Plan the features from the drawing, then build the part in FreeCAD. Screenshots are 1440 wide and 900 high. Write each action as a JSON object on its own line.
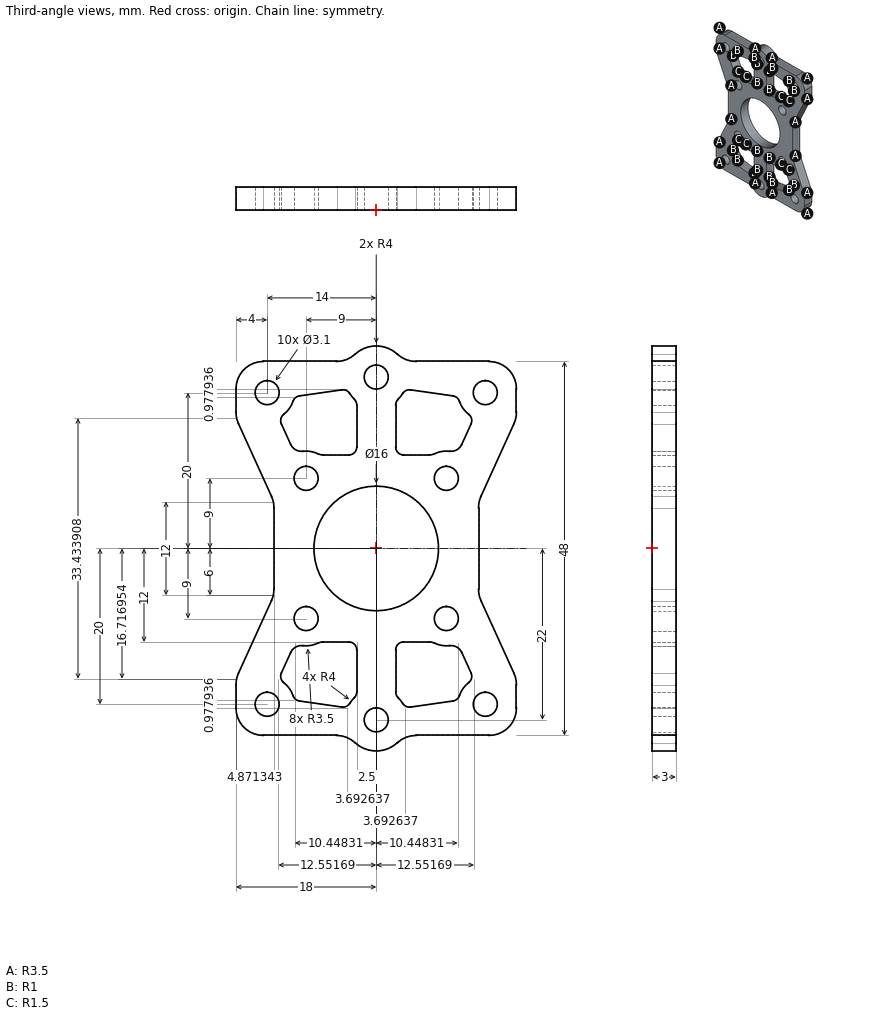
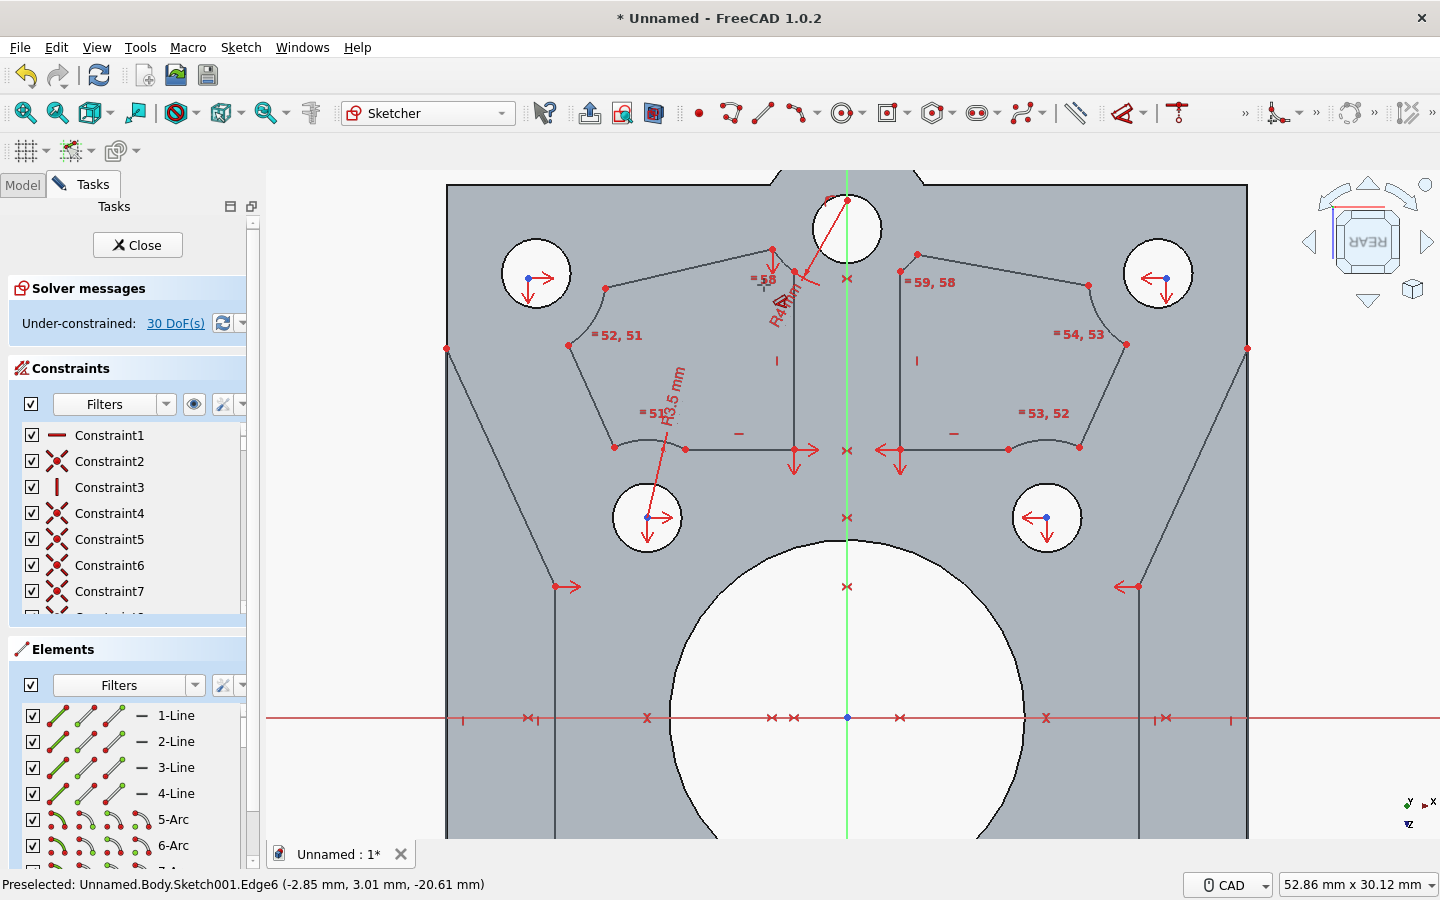
{"action": "left_click", "coordinate": [555, 774]}
{"action": "left_click", "coordinate": [521, 699]}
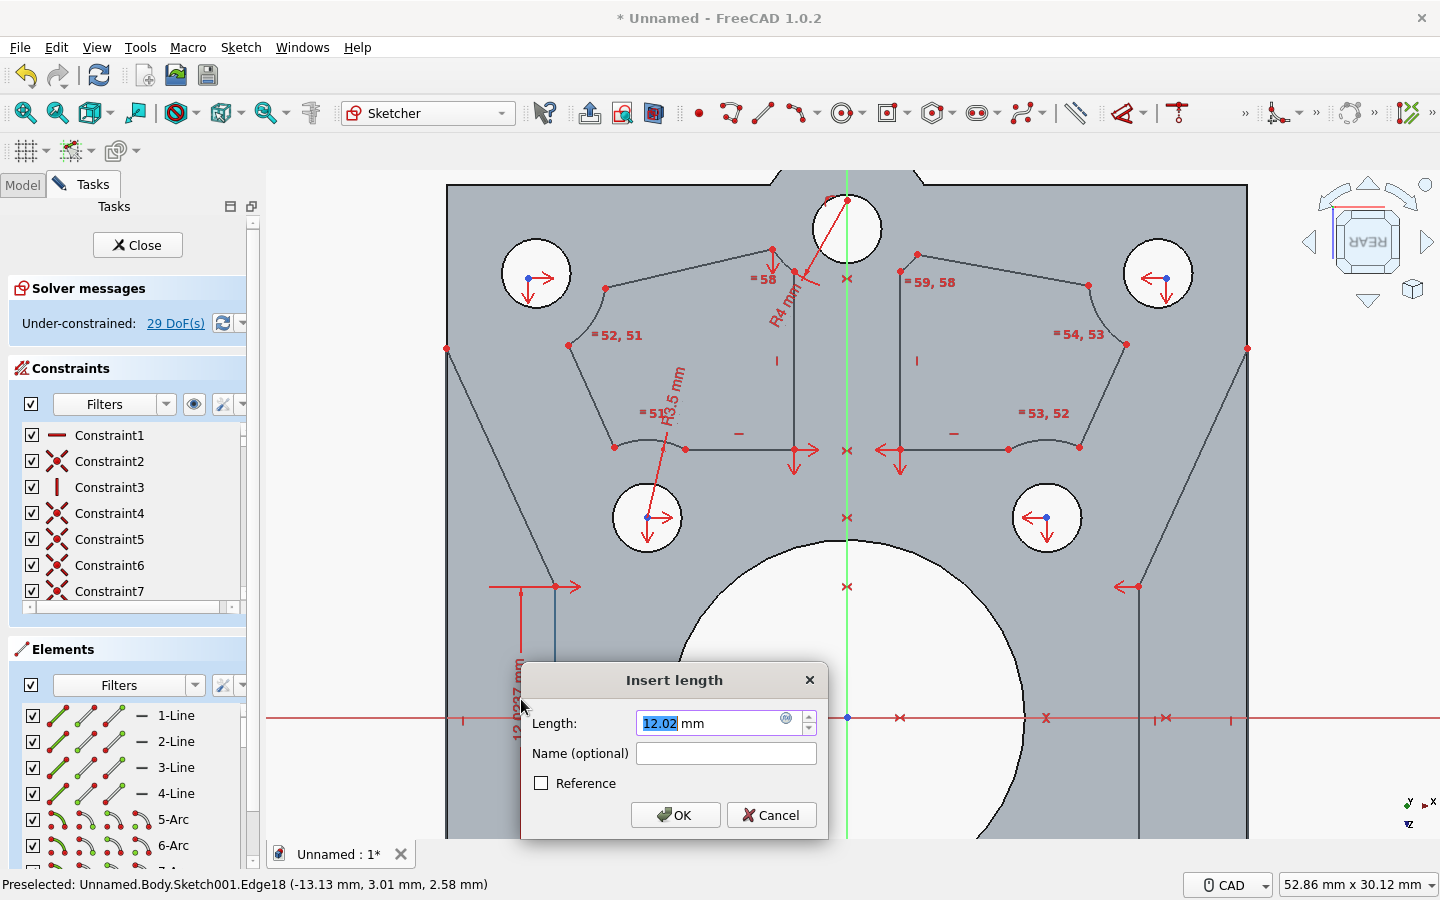
{"action": "type", "text": "12"}
{"action": "key", "text": "Return"}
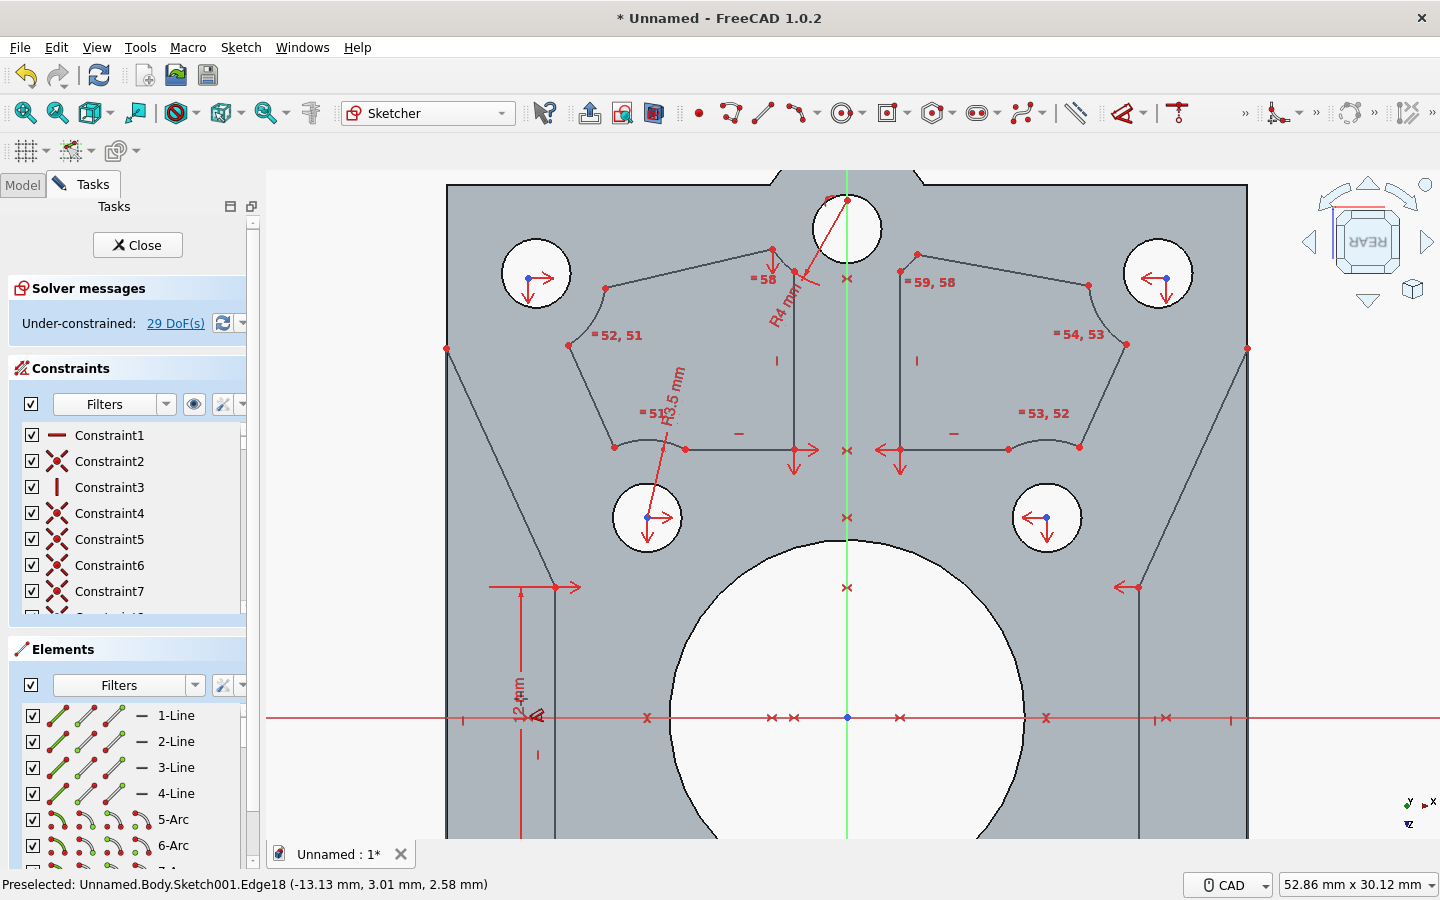
{"action": "left_click", "coordinate": [1139, 667]}
{"action": "left_click", "coordinate": [1173, 699]}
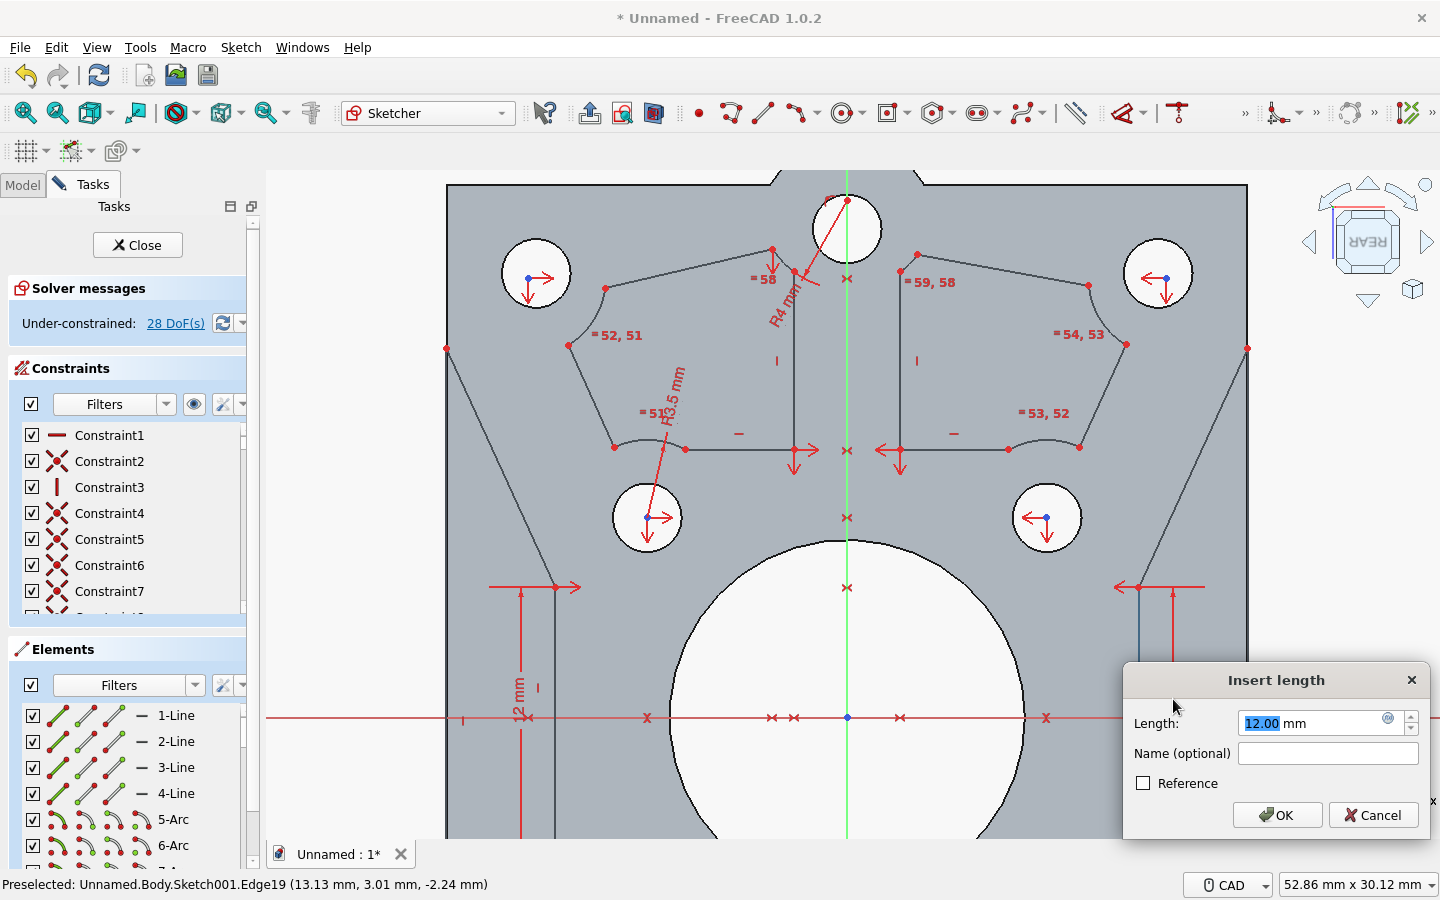
{"action": "type", "text": "12"}
{"action": "key", "text": "Return"}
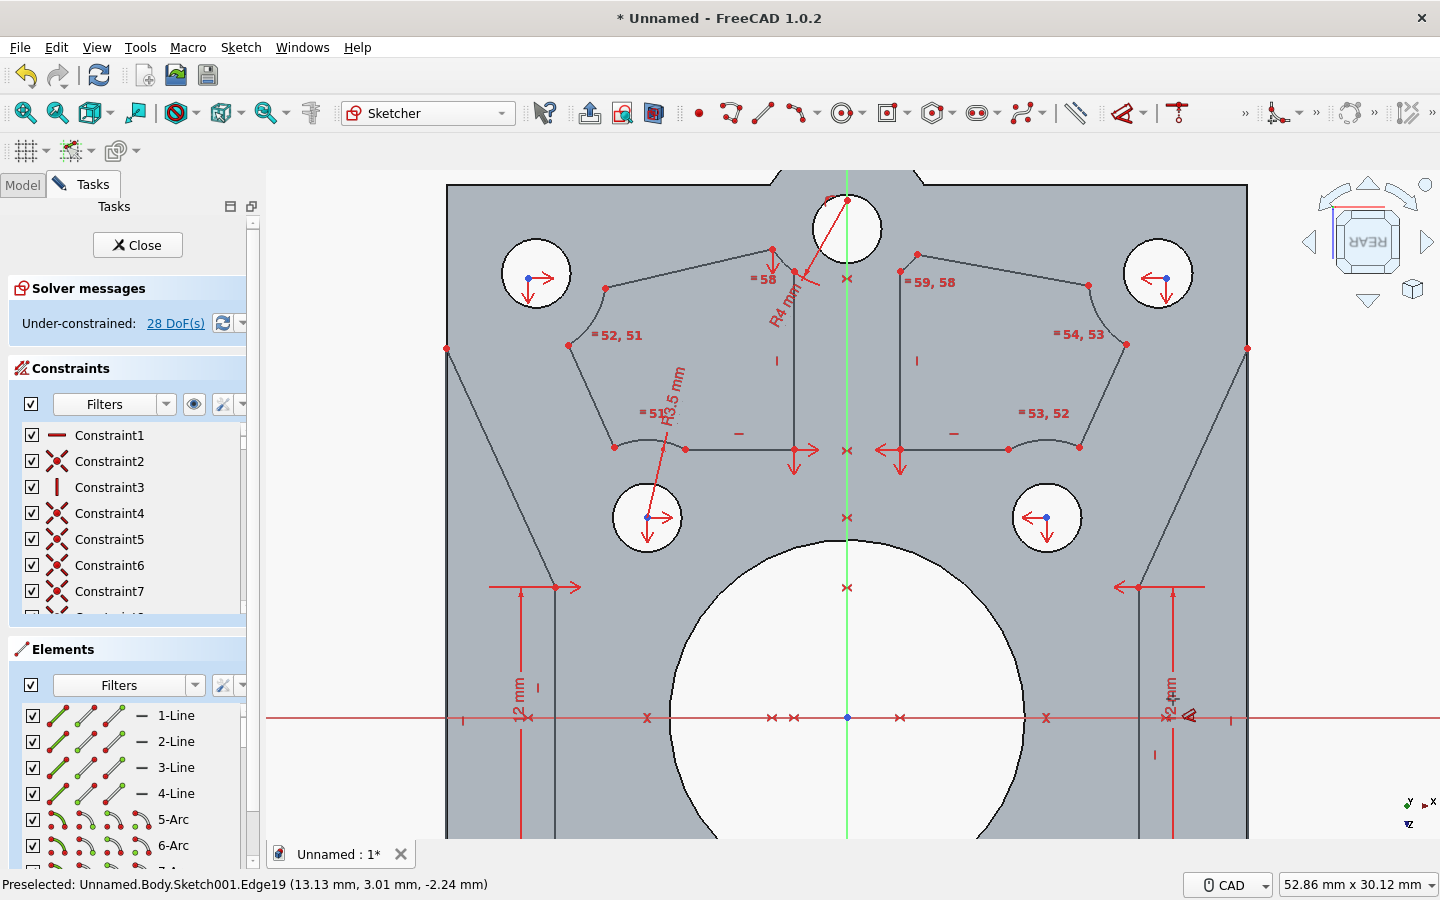
{"action": "left_click", "coordinate": [555, 587]}
{"action": "left_click", "coordinate": [521, 653]}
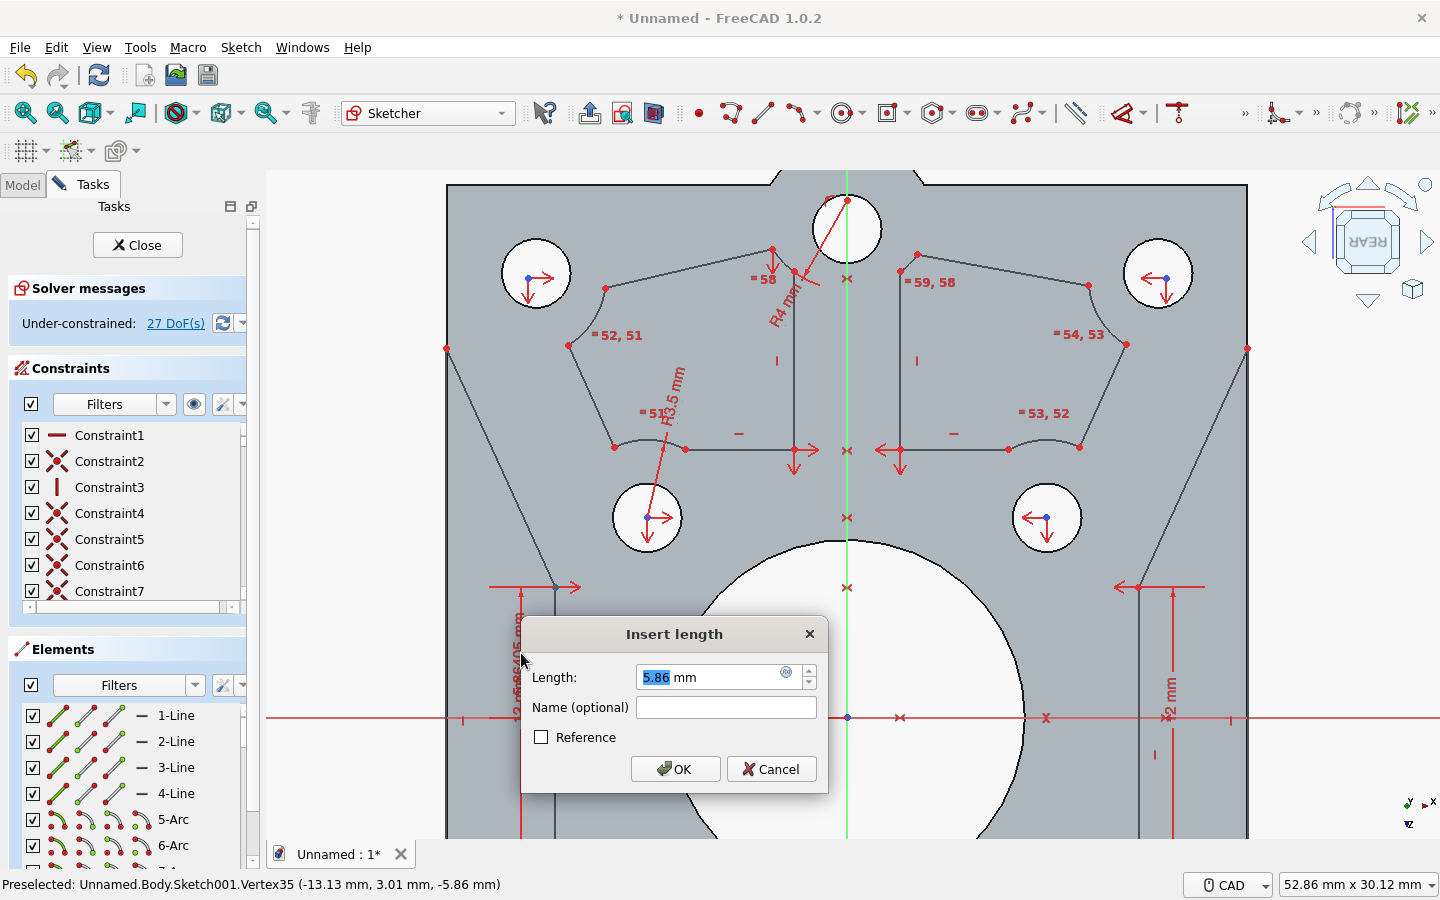
{"action": "type", "text": "6"}
{"action": "key", "text": "Return"}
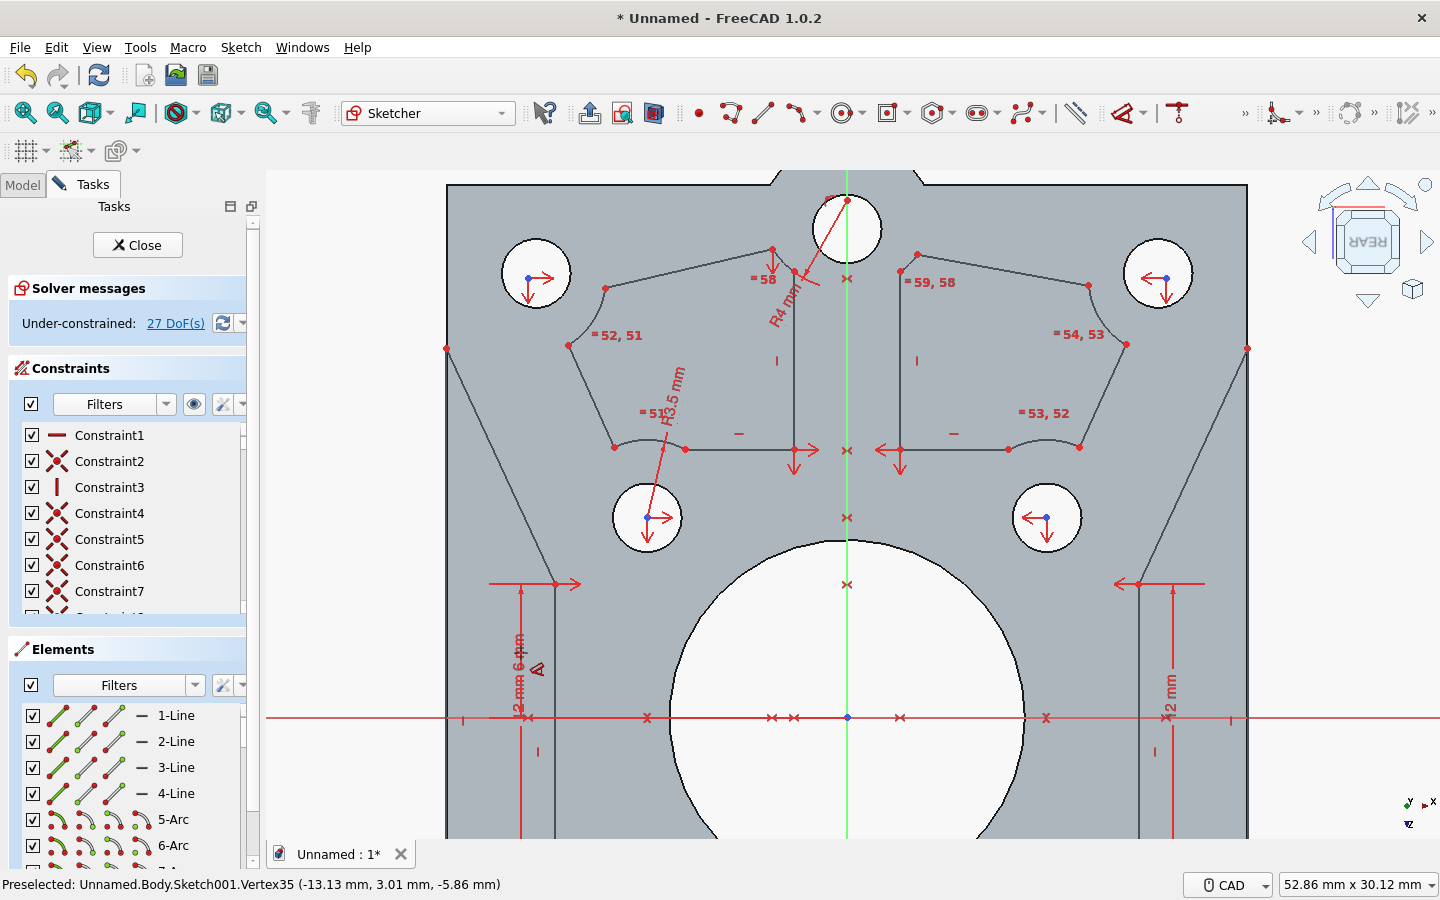
{"action": "left_click", "coordinate": [647, 518]}
{"action": "left_click", "coordinate": [747, 484]}